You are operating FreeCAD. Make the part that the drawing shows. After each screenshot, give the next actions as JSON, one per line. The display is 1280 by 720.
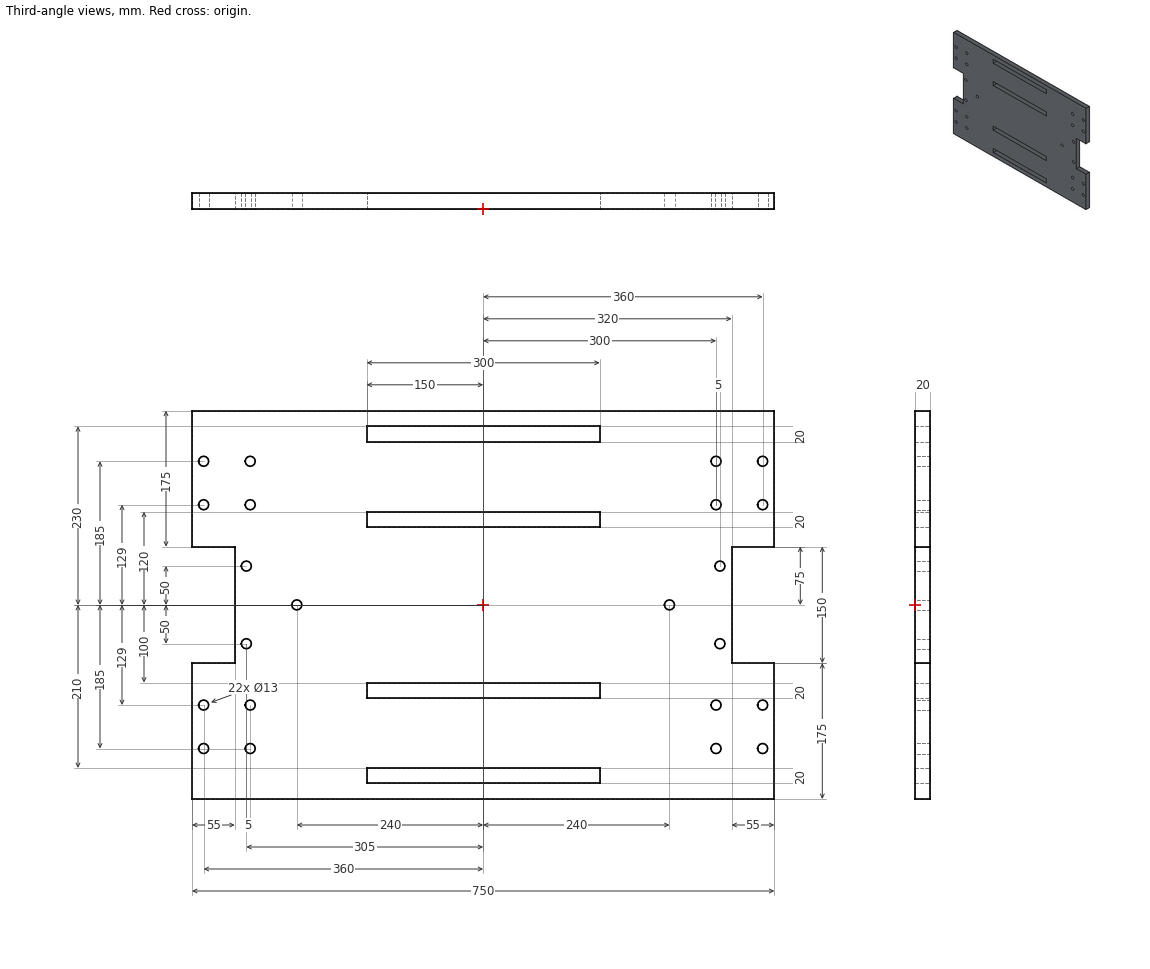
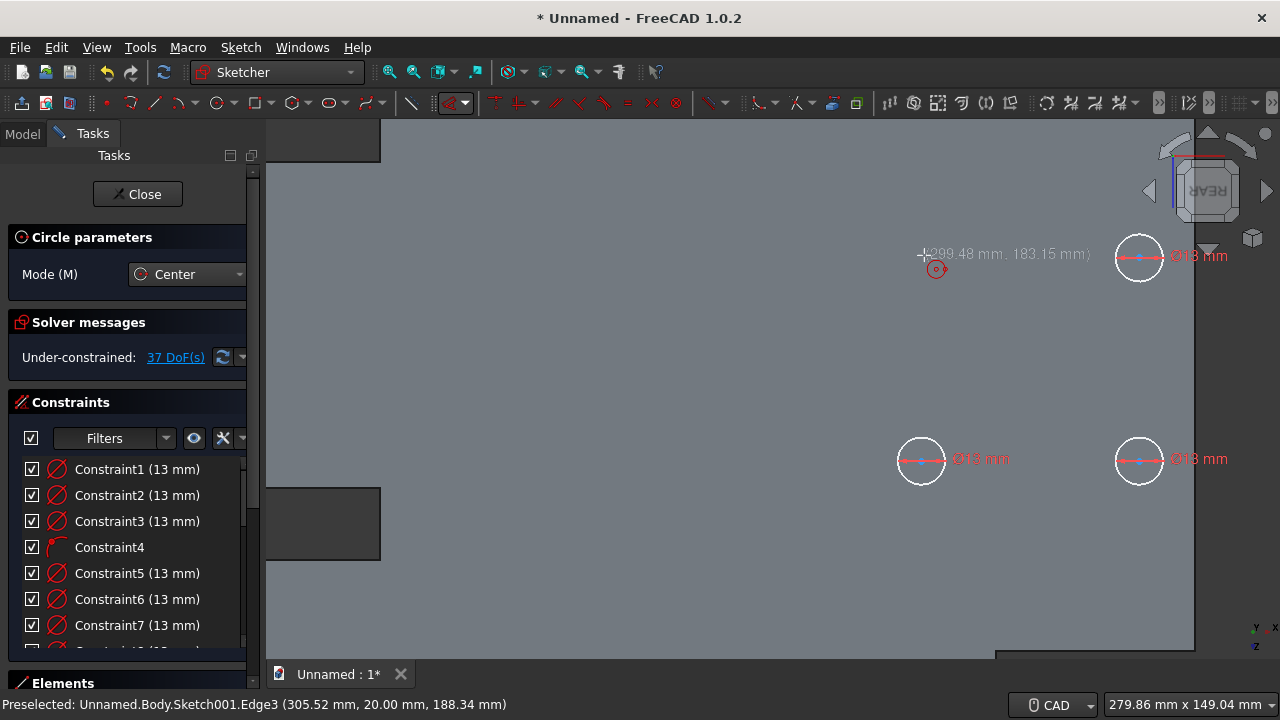
{"action": "scroll", "coordinate": [924, 254], "scroll_direction": "down", "scroll_amount": 8}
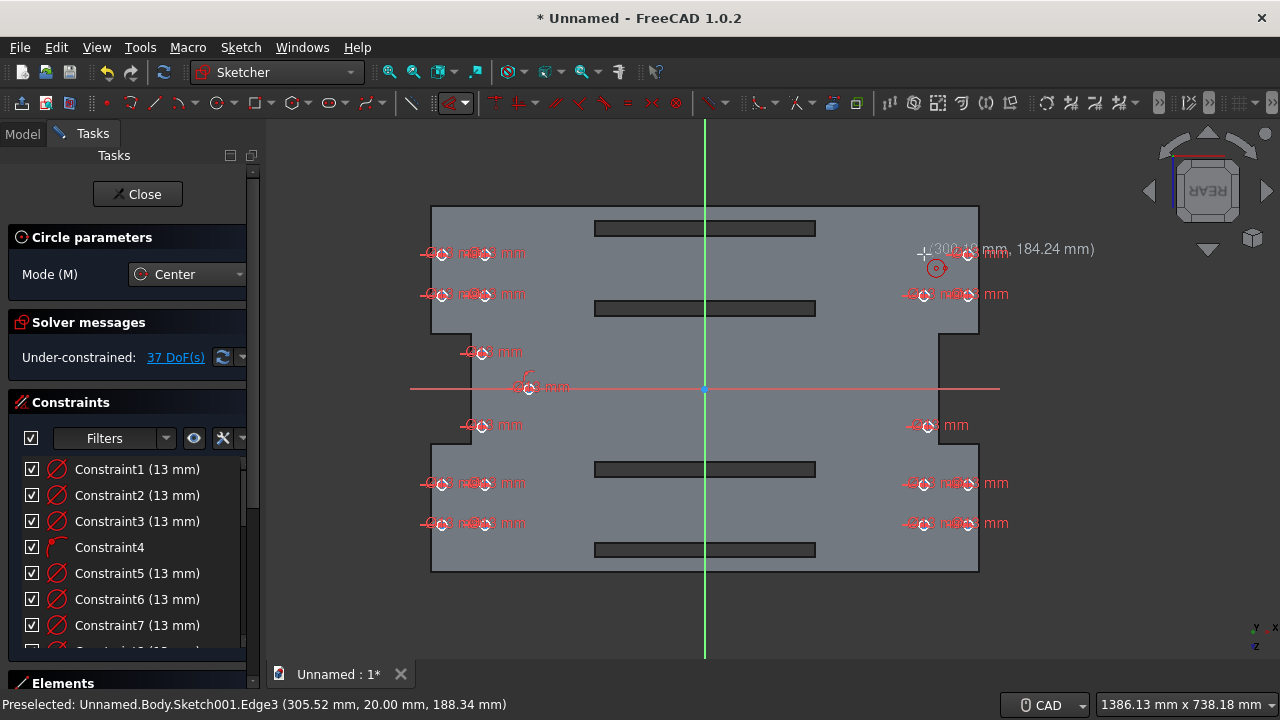
{"action": "left_click", "coordinate": [924, 254]}
{"action": "mouse_move", "coordinate": [928, 250]}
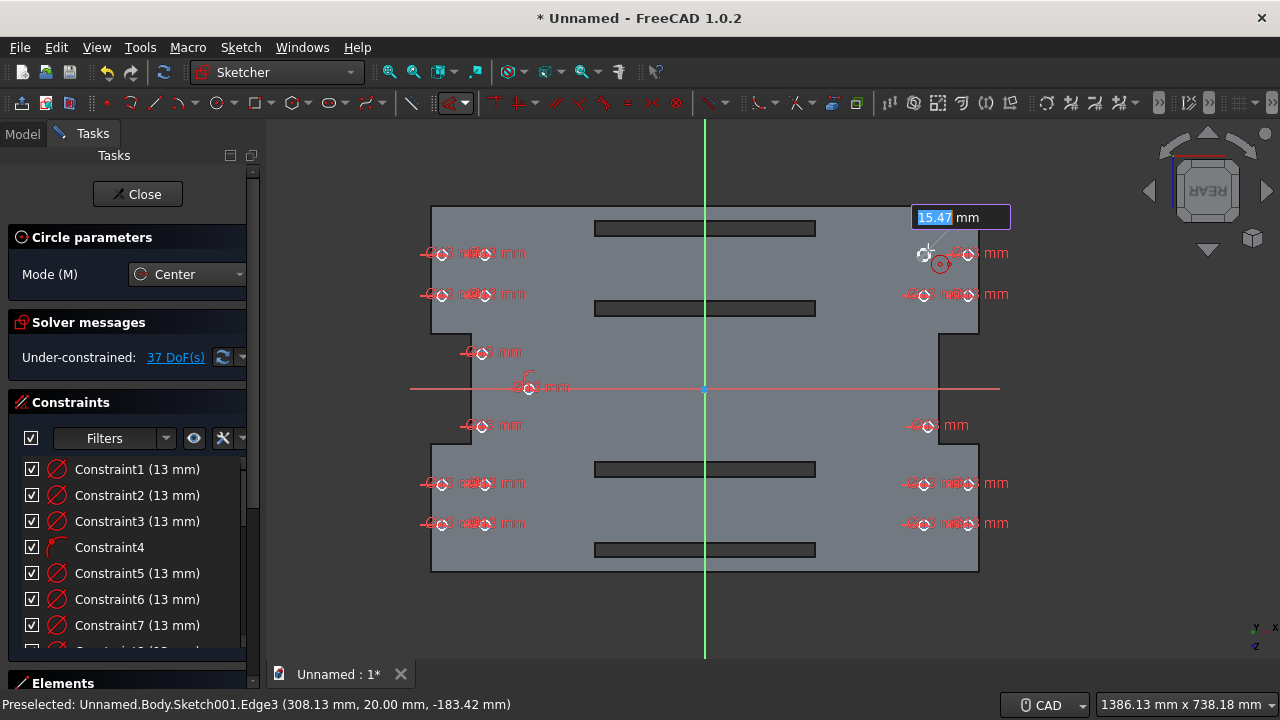
{"action": "type", "text": "13"}
{"action": "key", "text": "Return"}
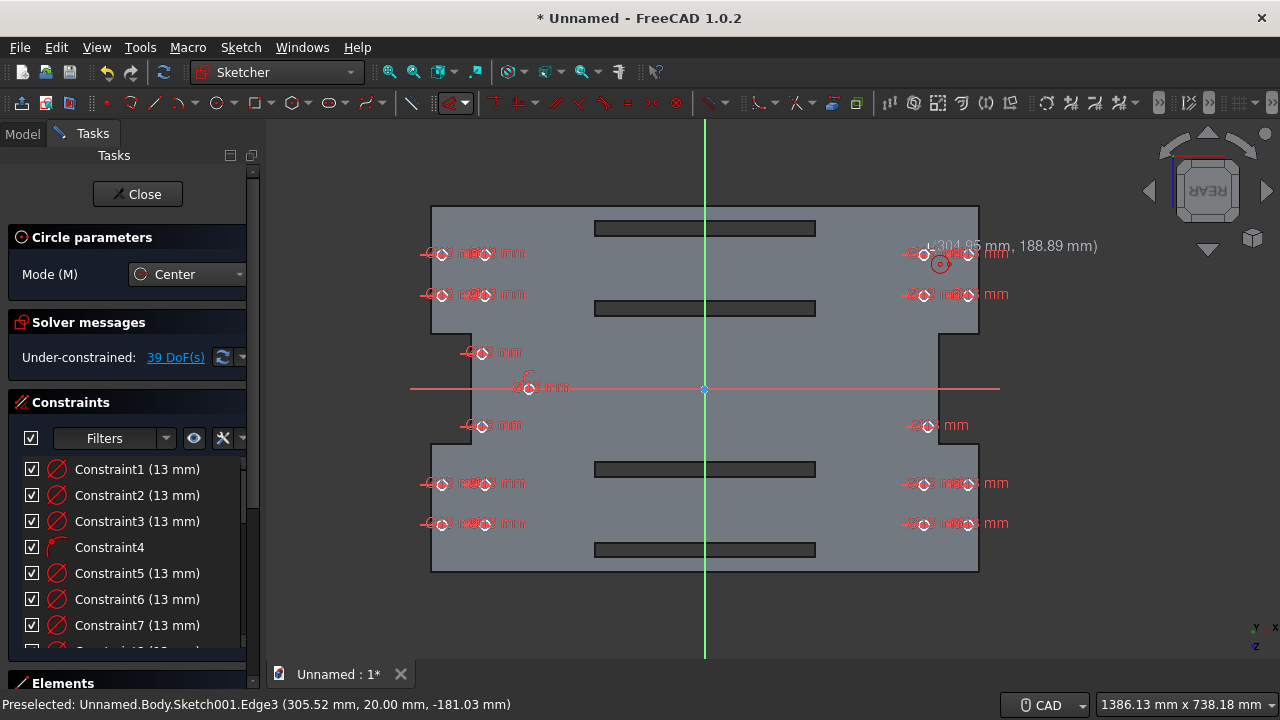
{"action": "scroll", "coordinate": [880, 389], "scroll_direction": "up", "scroll_amount": 8}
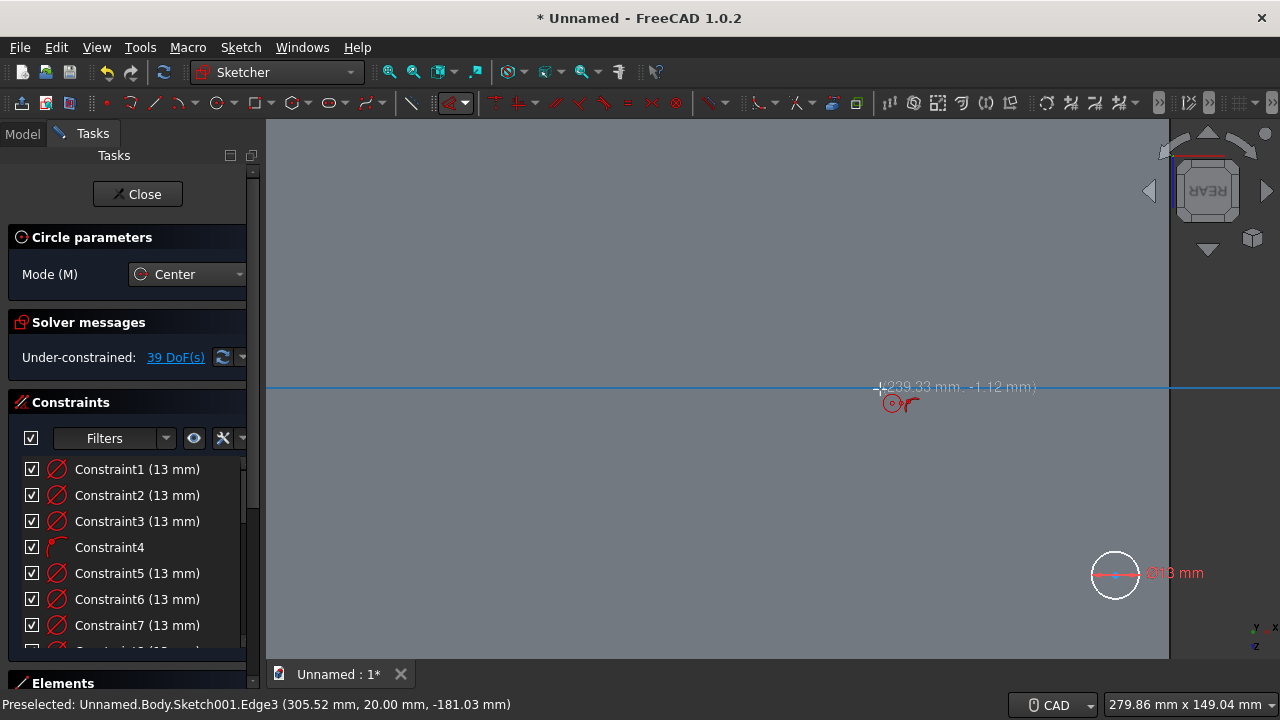
{"action": "scroll", "coordinate": [880, 389], "scroll_direction": "down", "scroll_amount": 8}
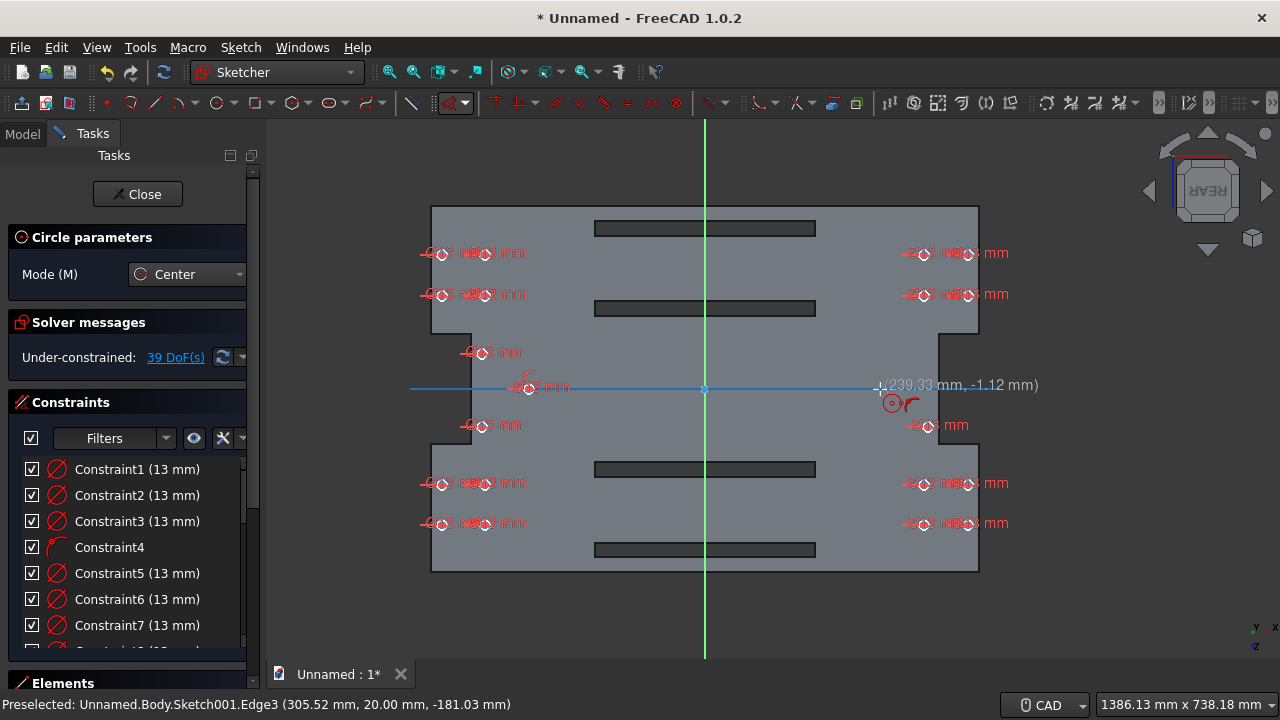
{"action": "left_click", "coordinate": [880, 389]}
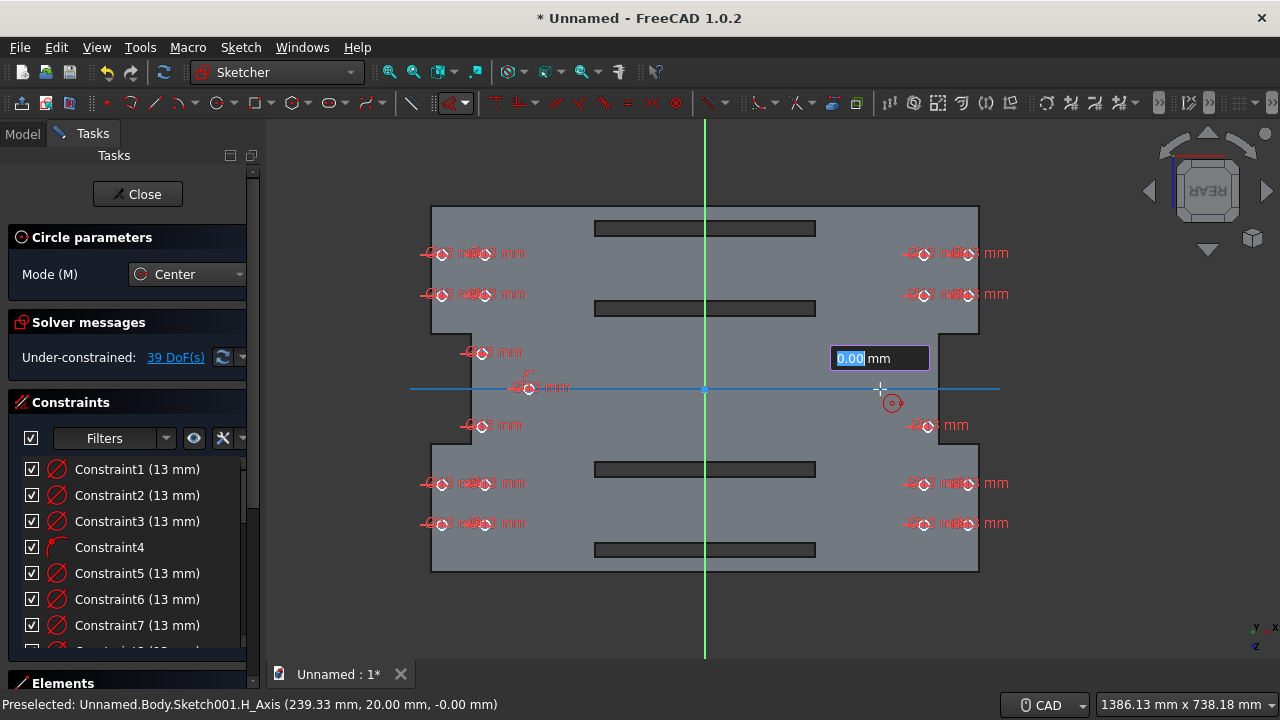
{"action": "scroll", "coordinate": [879, 394], "scroll_direction": "up", "scroll_amount": 7}
{"action": "mouse_move", "coordinate": [877, 391]}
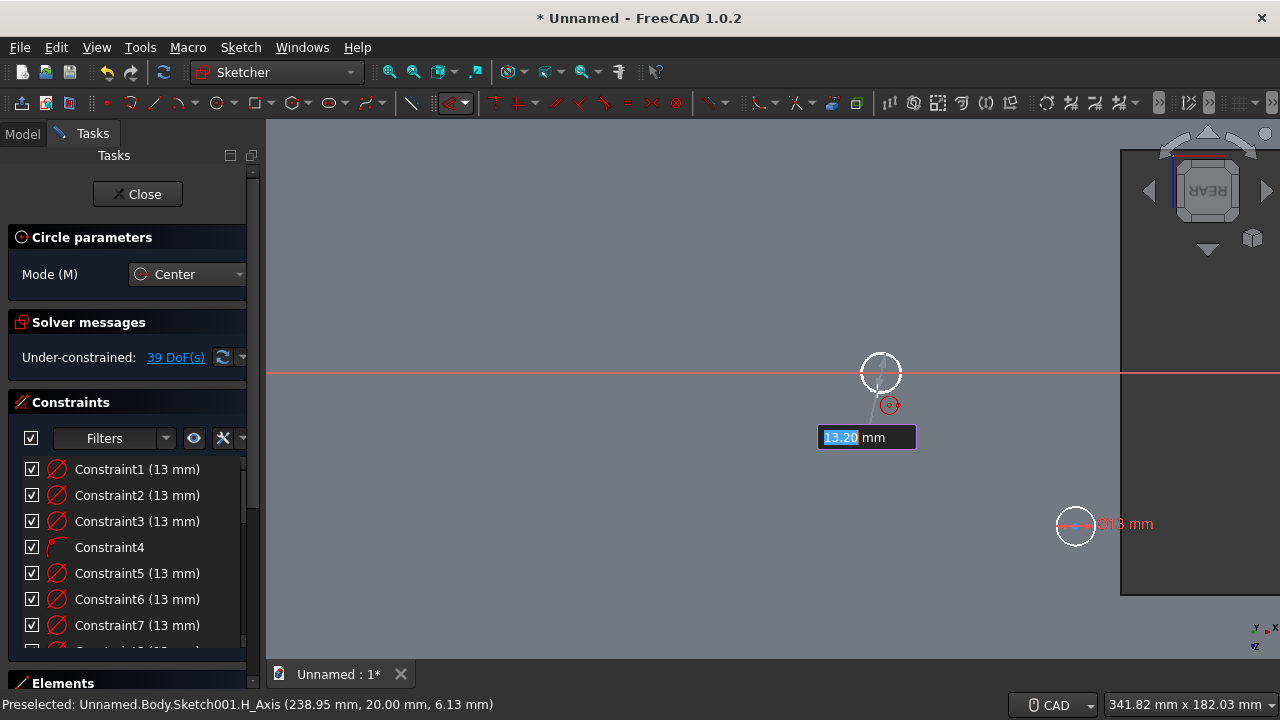
{"action": "type", "text": "13"}
{"action": "key", "text": "Return"}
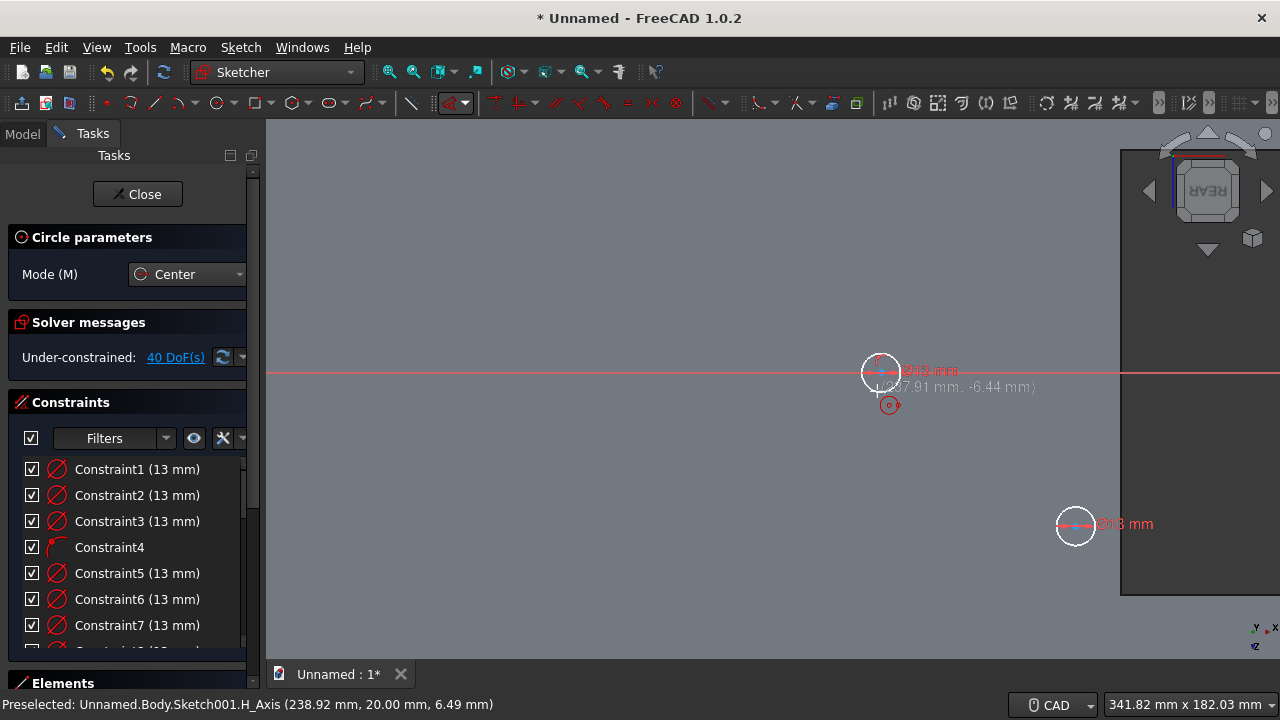
{"action": "scroll", "coordinate": [879, 394], "scroll_direction": "down", "scroll_amount": 7}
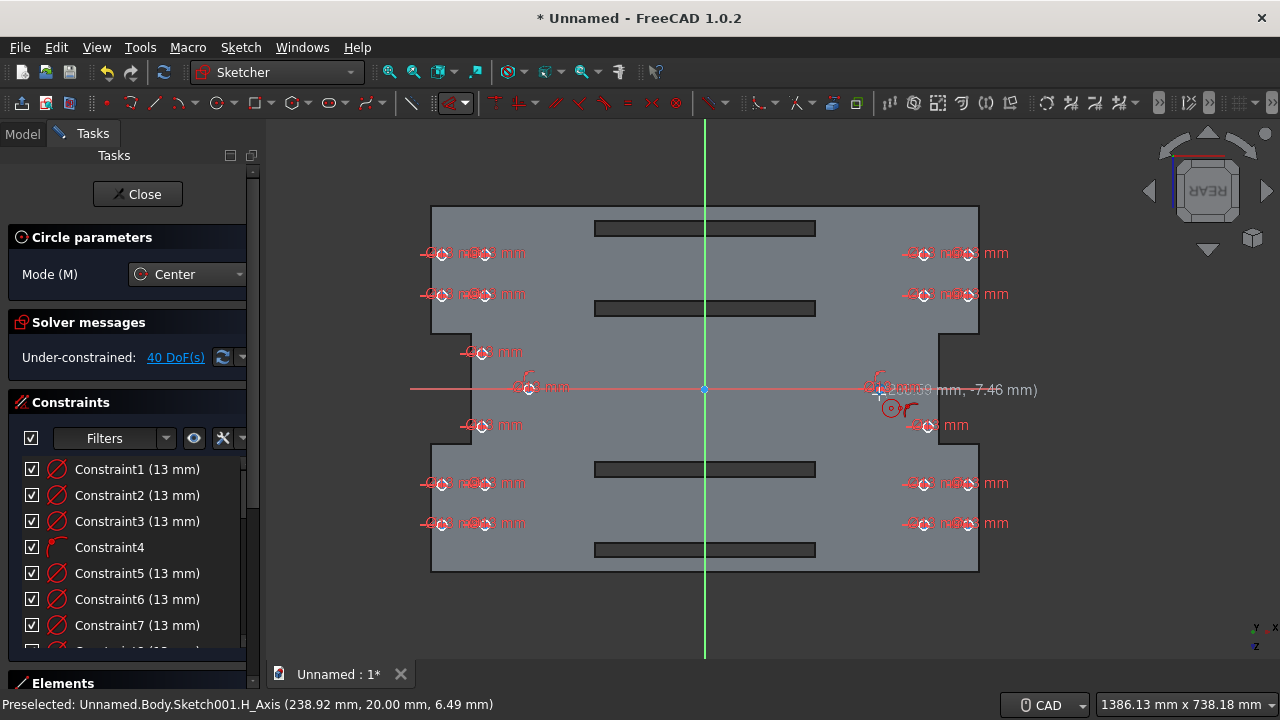
{"action": "left_click", "coordinate": [928, 353]}
{"action": "mouse_move", "coordinate": [931, 349]}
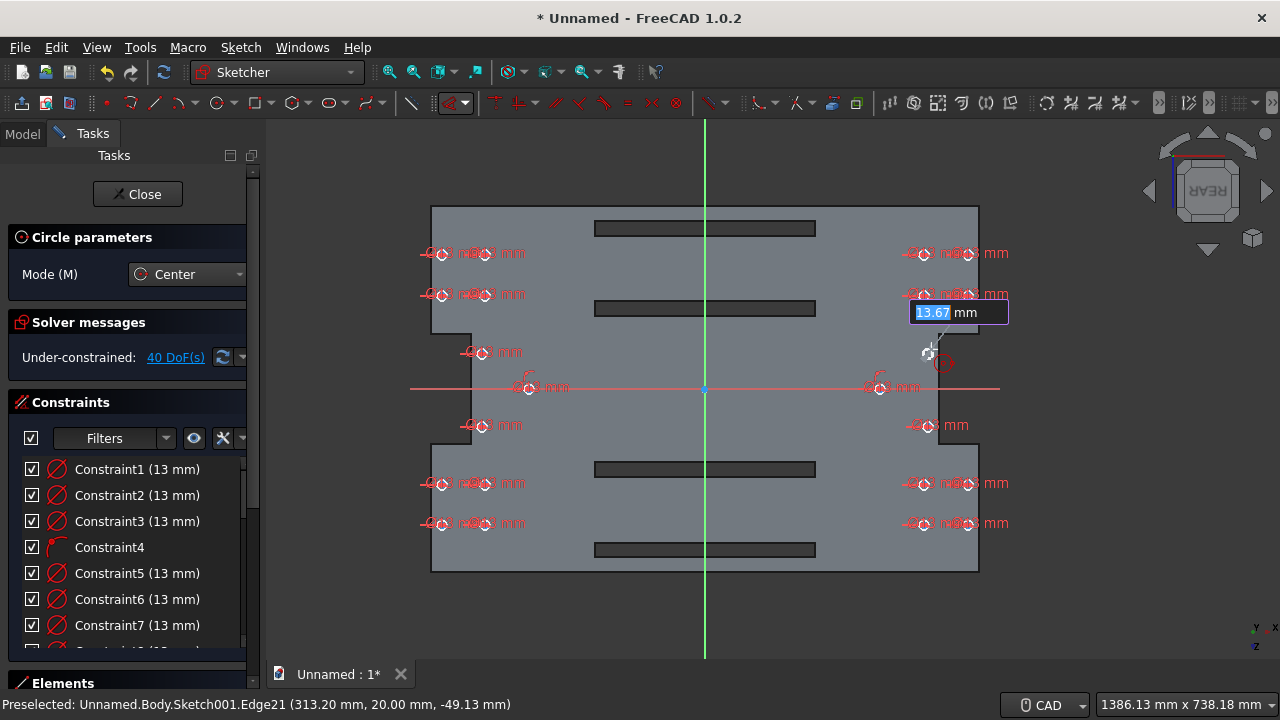
{"action": "type", "text": "13"}
{"action": "key", "text": "Return"}
{"action": "key", "text": "Escape"}